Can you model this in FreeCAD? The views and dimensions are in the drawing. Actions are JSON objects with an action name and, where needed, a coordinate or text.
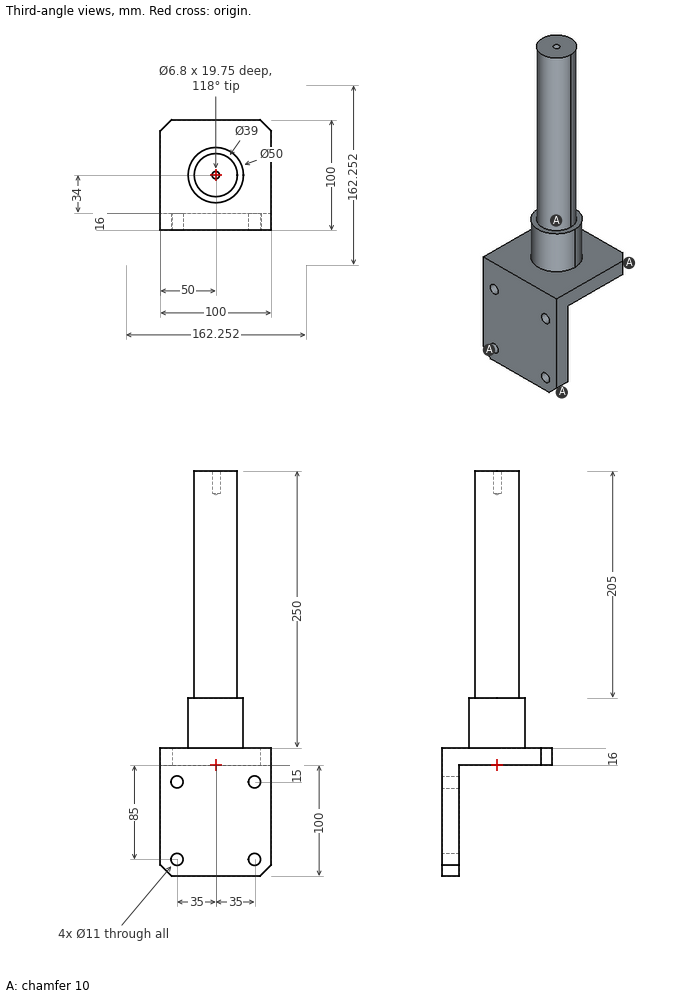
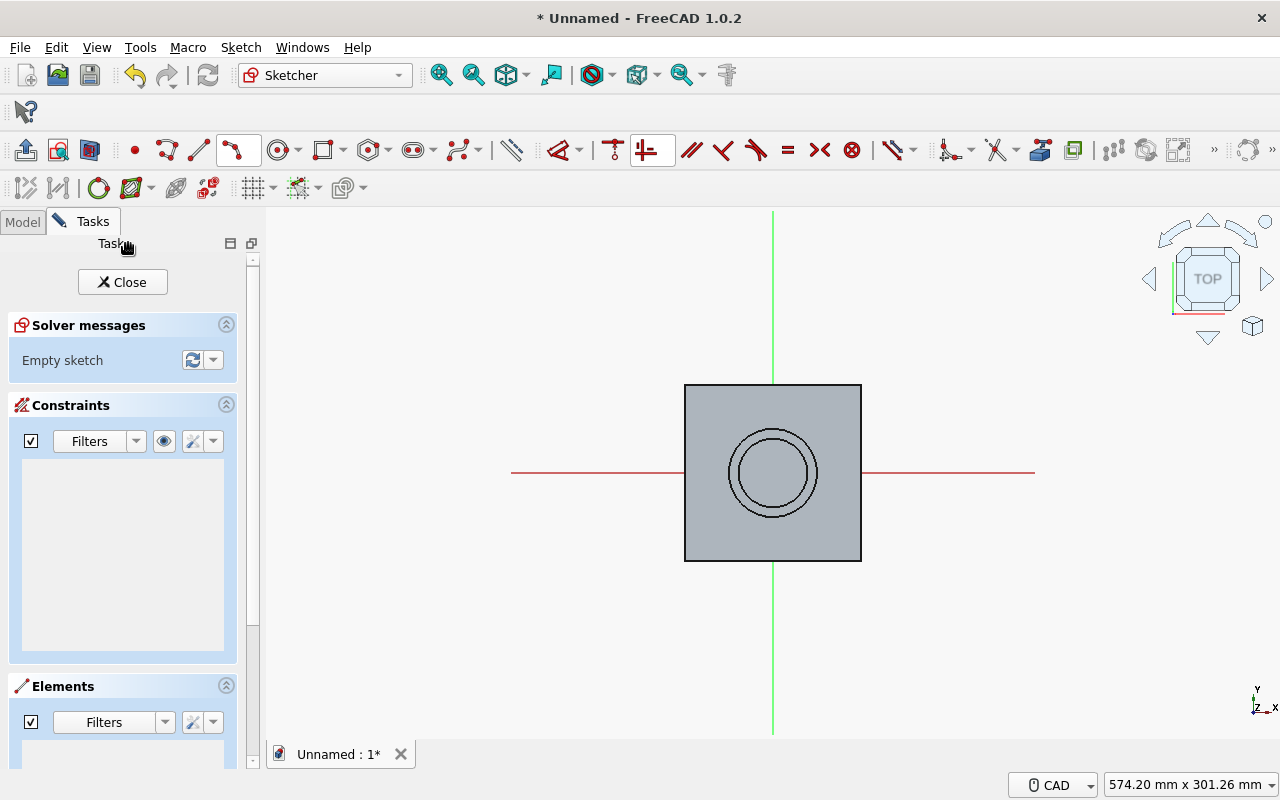
{"action": "left_click", "coordinate": [90, 150]}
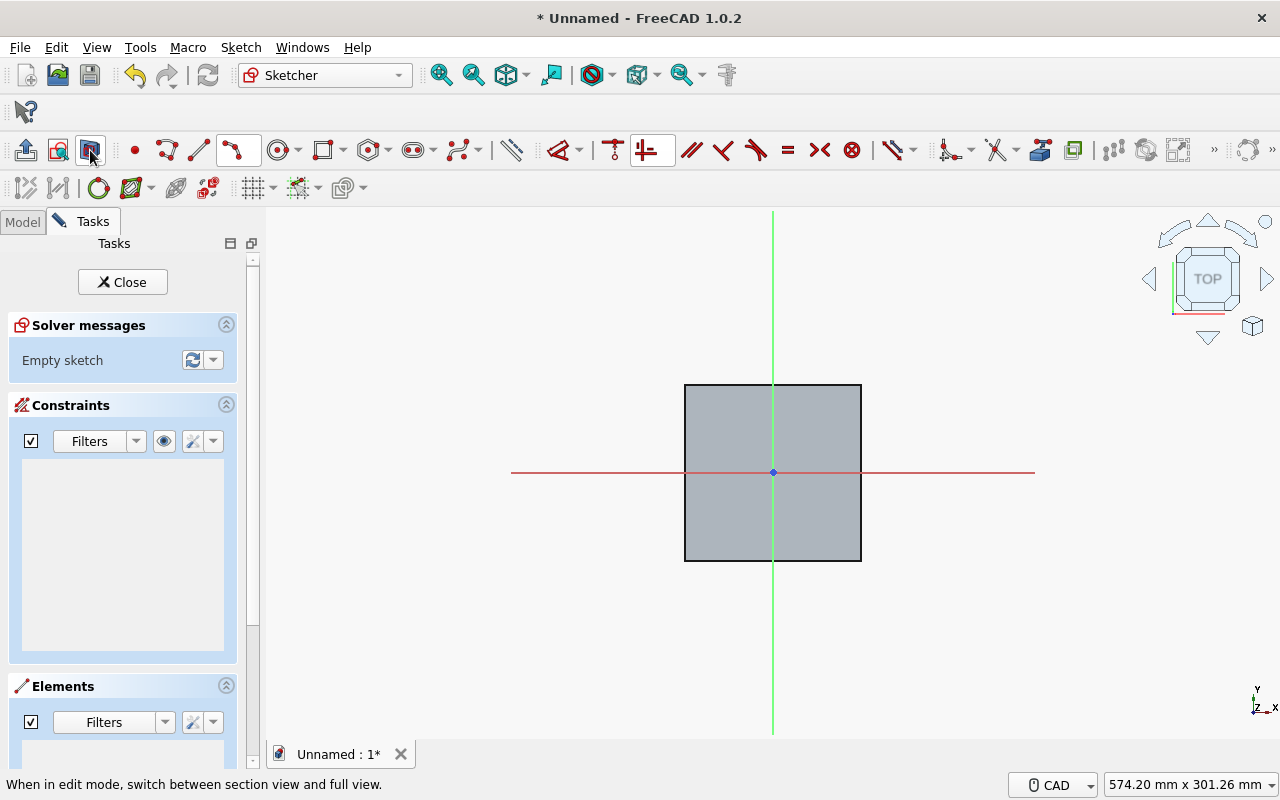
{"action": "scroll", "coordinate": [803, 536], "scroll_direction": "up", "scroll_amount": 6}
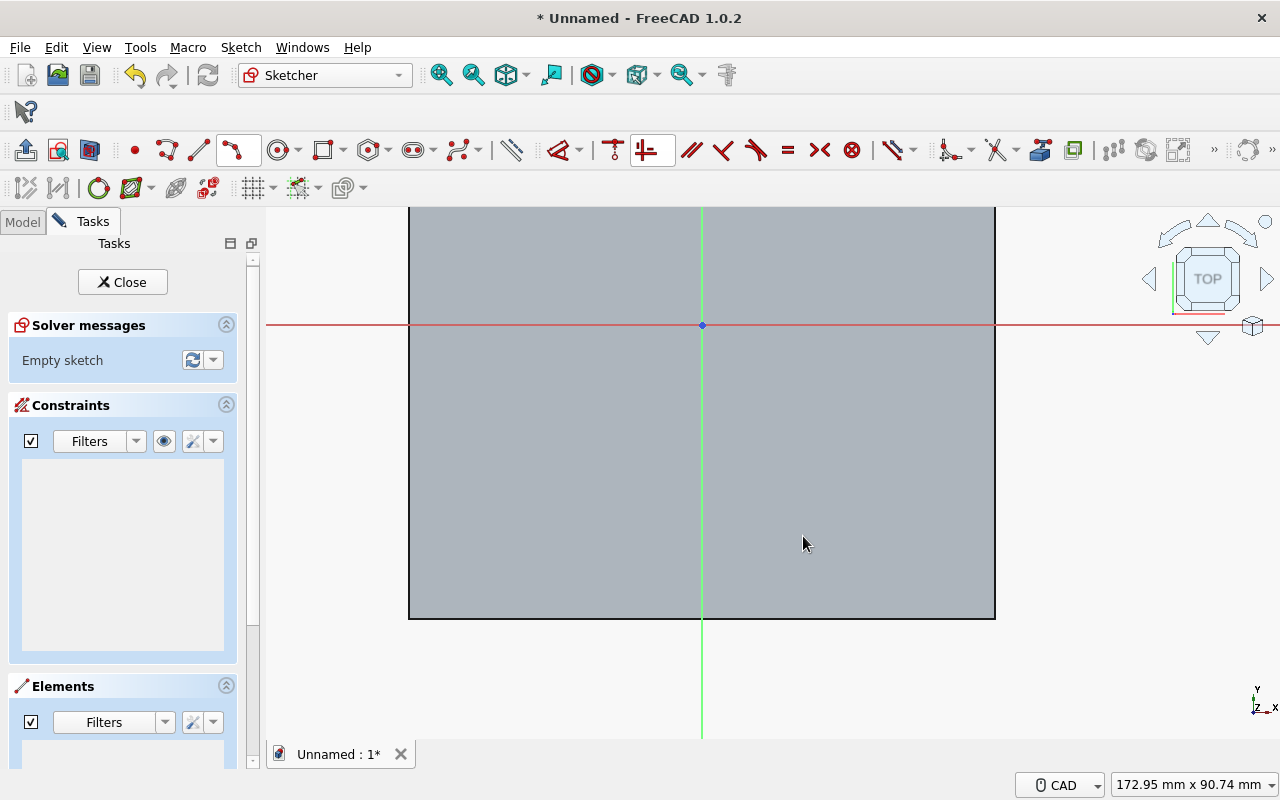
{"action": "key", "text": "g r"}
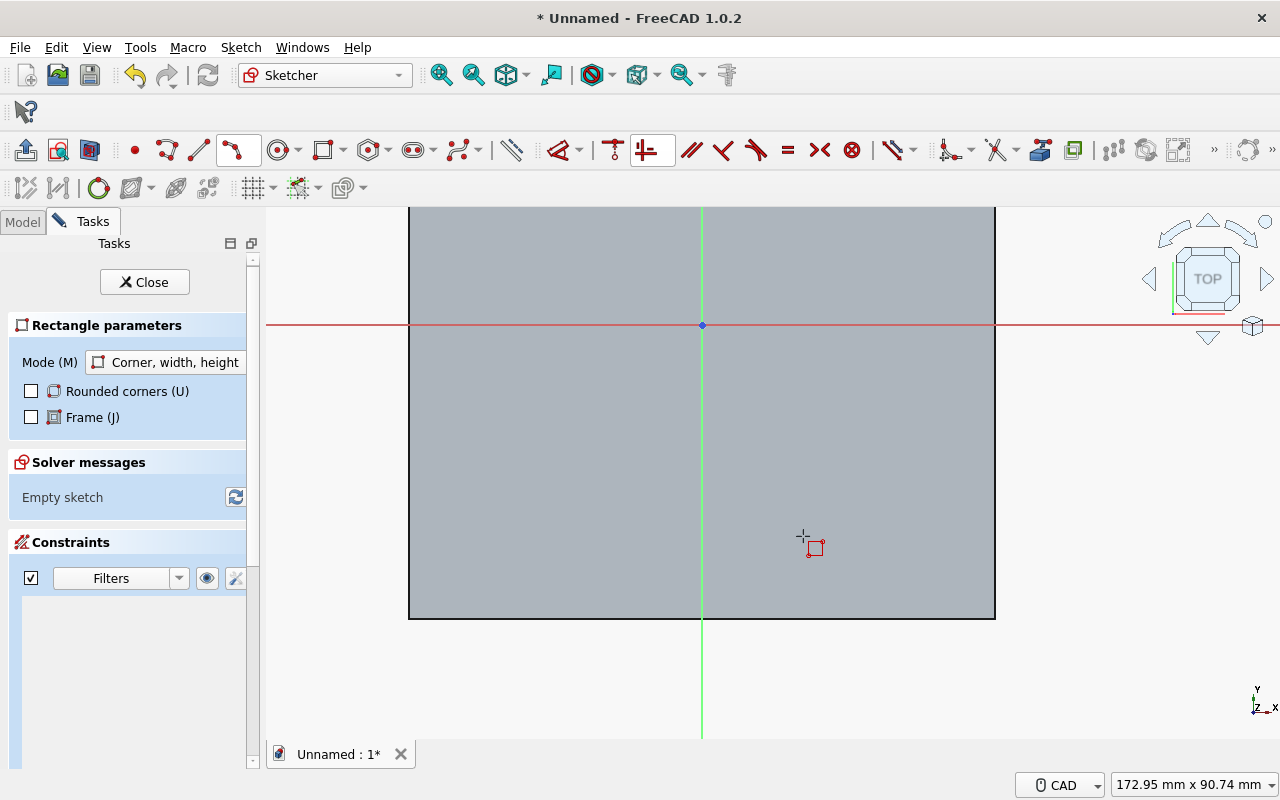
{"action": "left_click", "coordinate": [409, 525]}
{"action": "left_click", "coordinate": [995, 619]}
{"action": "key", "text": "Escape"}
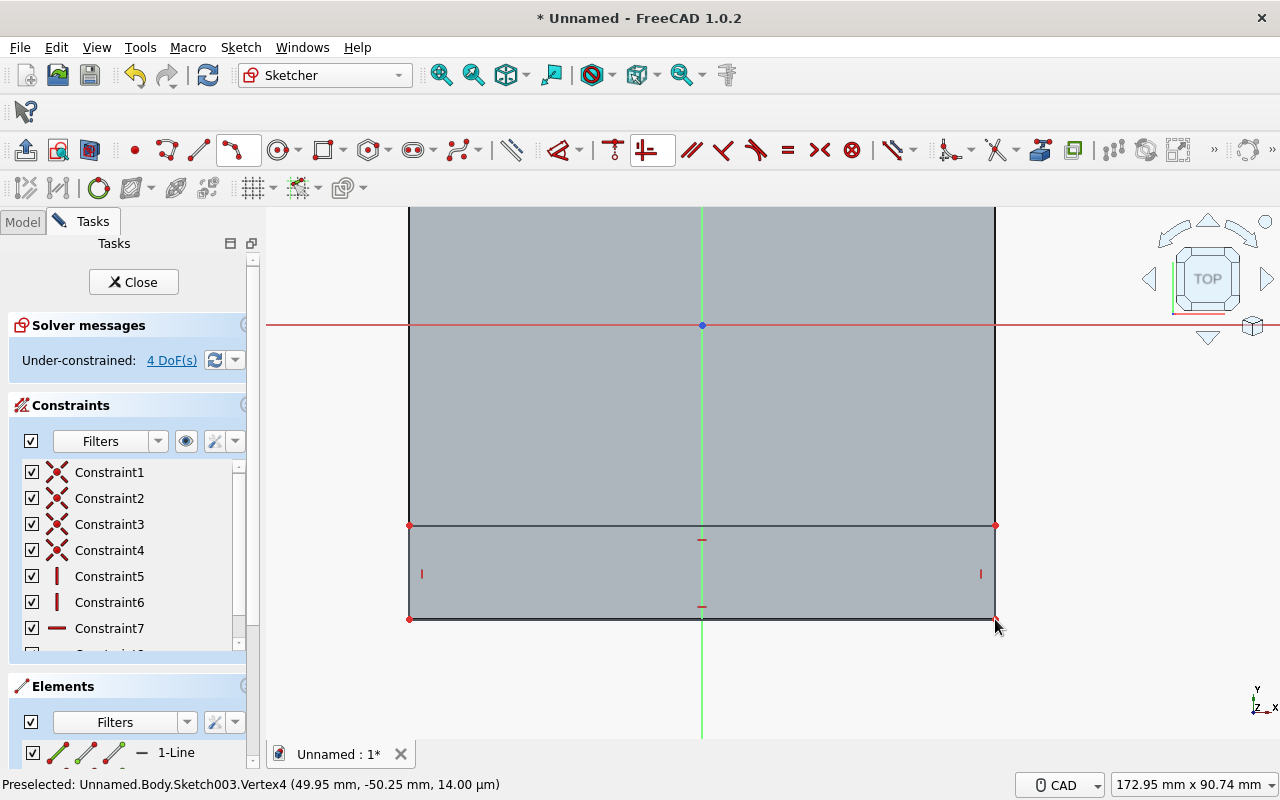
{"action": "key", "text": "d"}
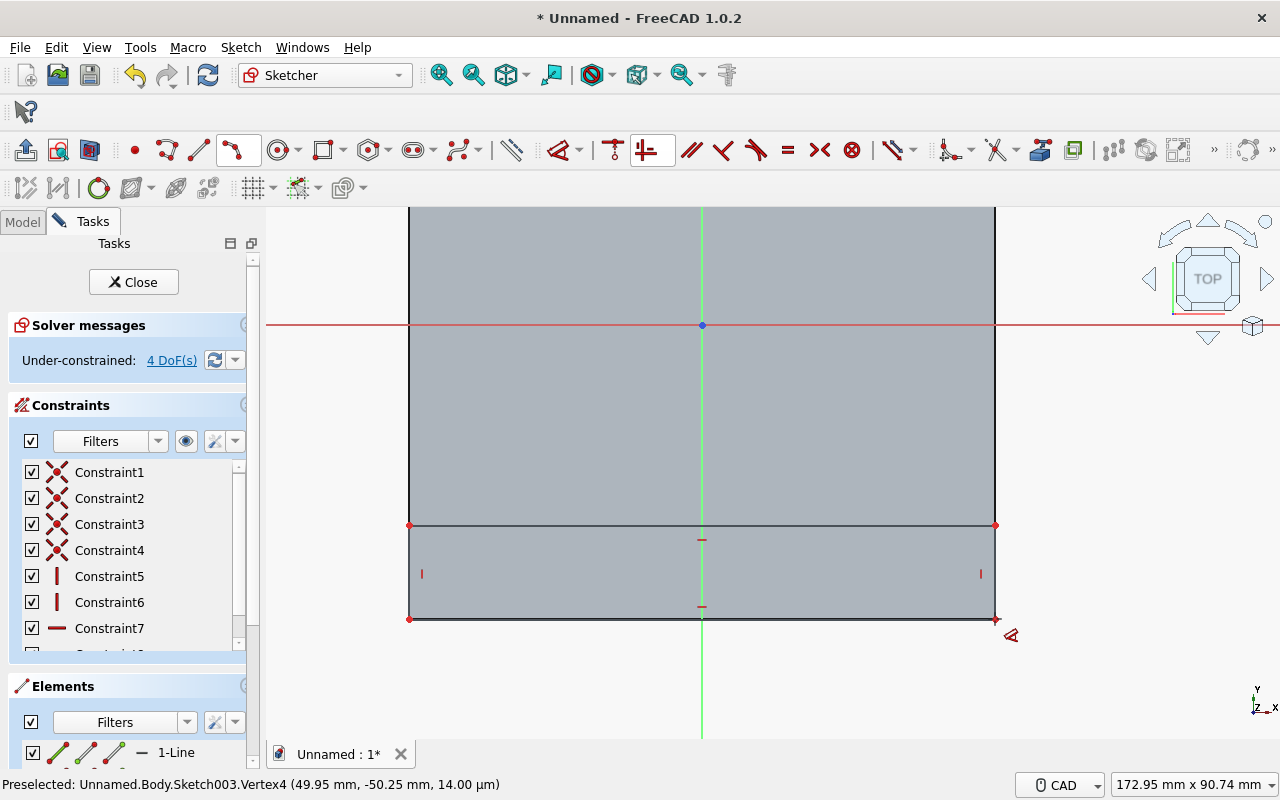
{"action": "left_click", "coordinate": [409, 554]}
{"action": "left_click", "coordinate": [375, 573]}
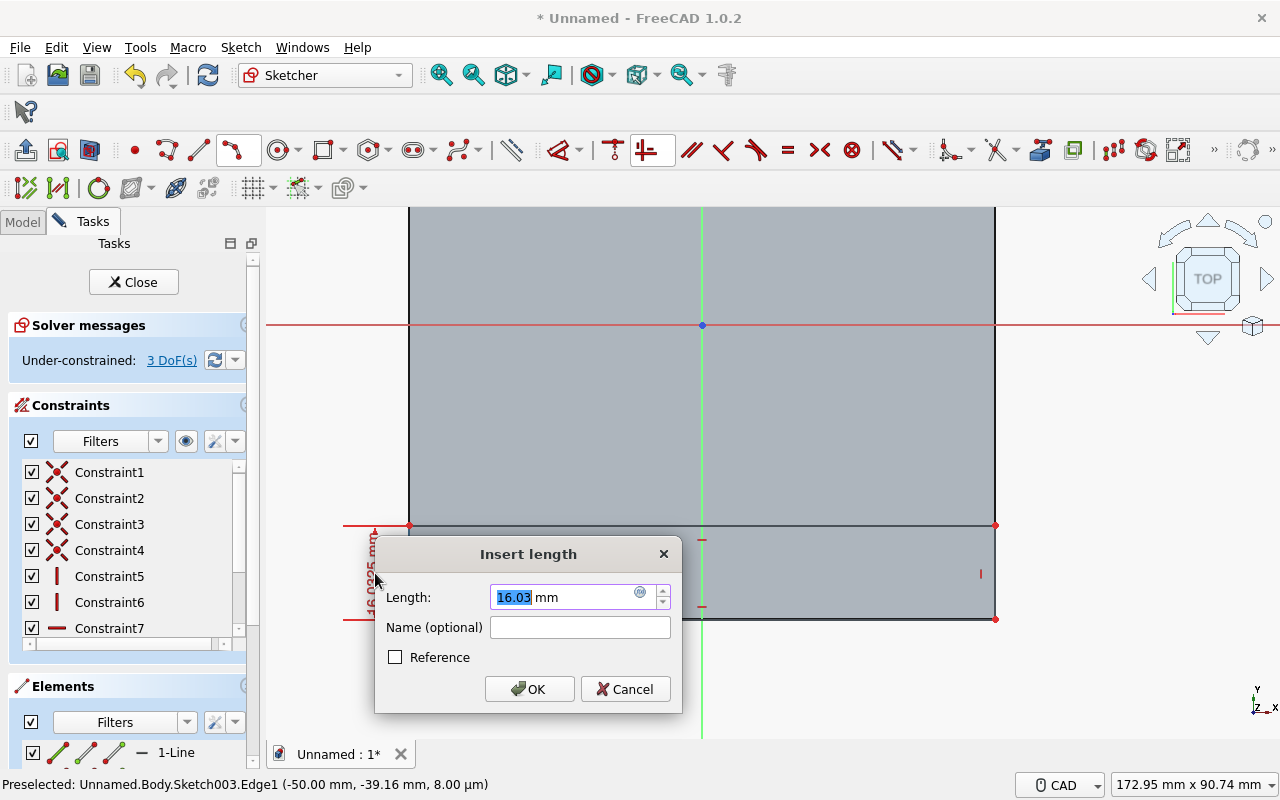
{"action": "type", "text": "16"}
{"action": "key", "text": "Return"}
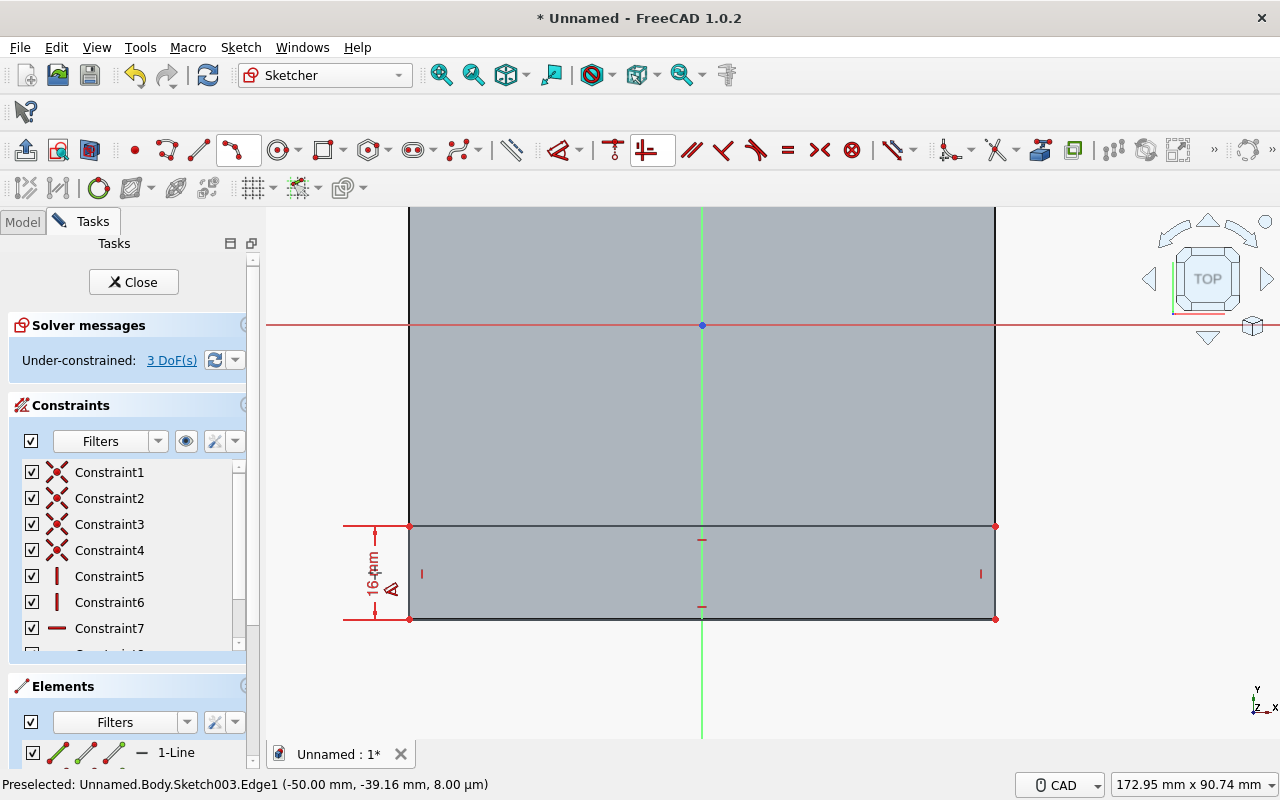
{"action": "left_click", "coordinate": [585, 620]}
{"action": "left_click", "coordinate": [567, 654]}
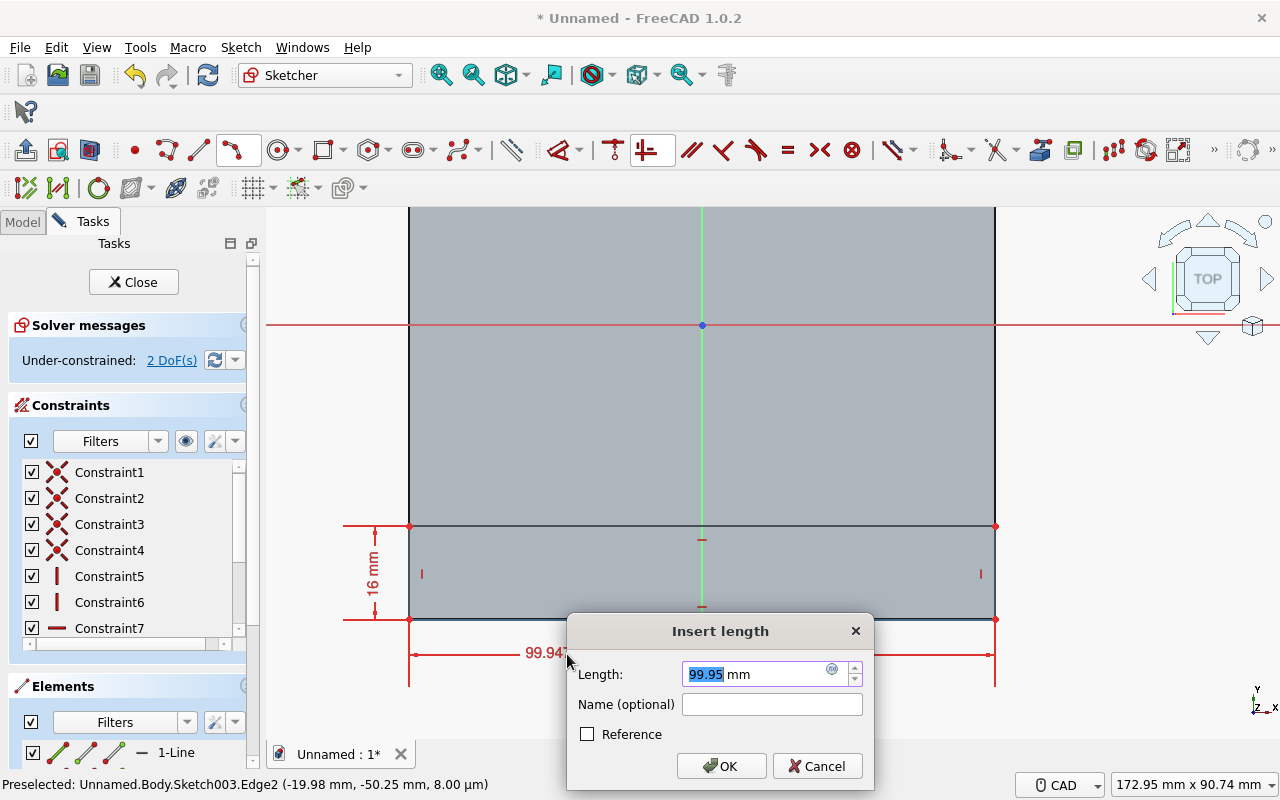
{"action": "type", "text": "100"}
{"action": "key", "text": "Return"}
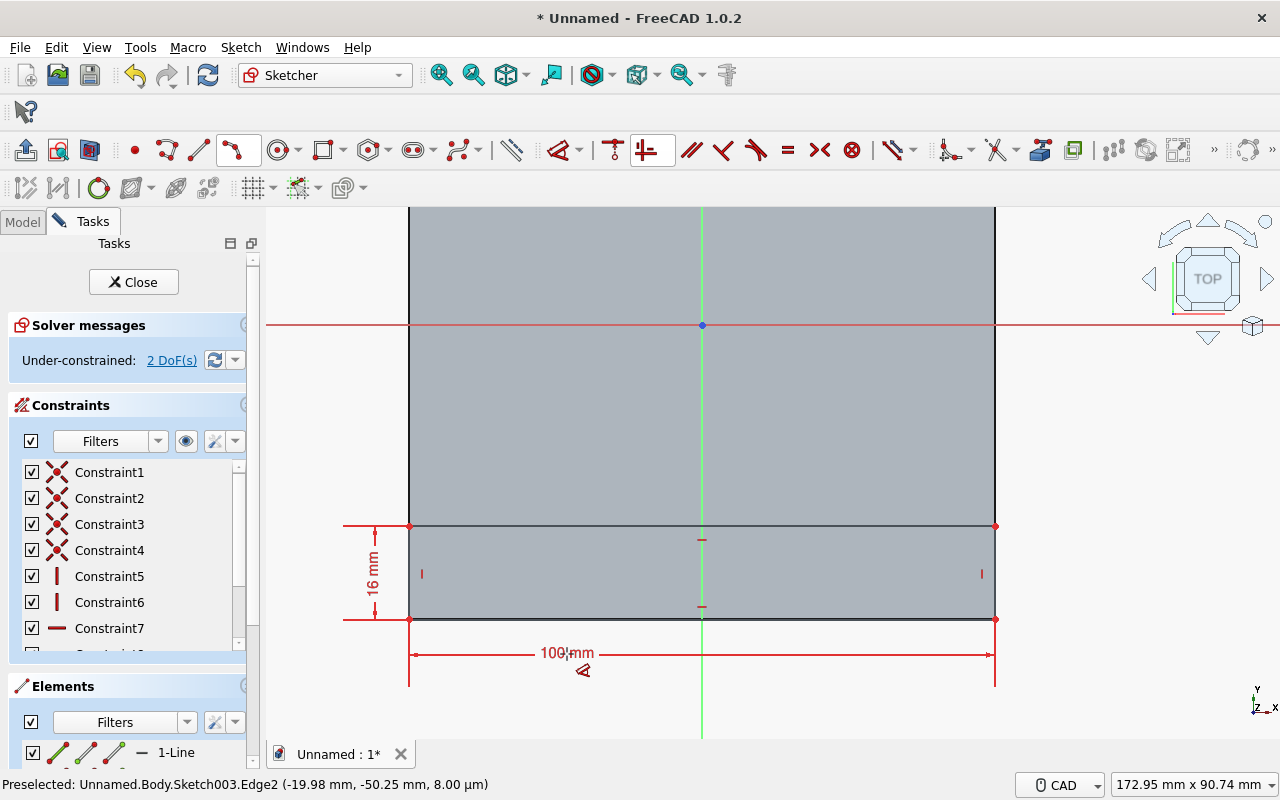
{"action": "left_click", "coordinate": [409, 526]}
{"action": "left_click", "coordinate": [556, 291]}